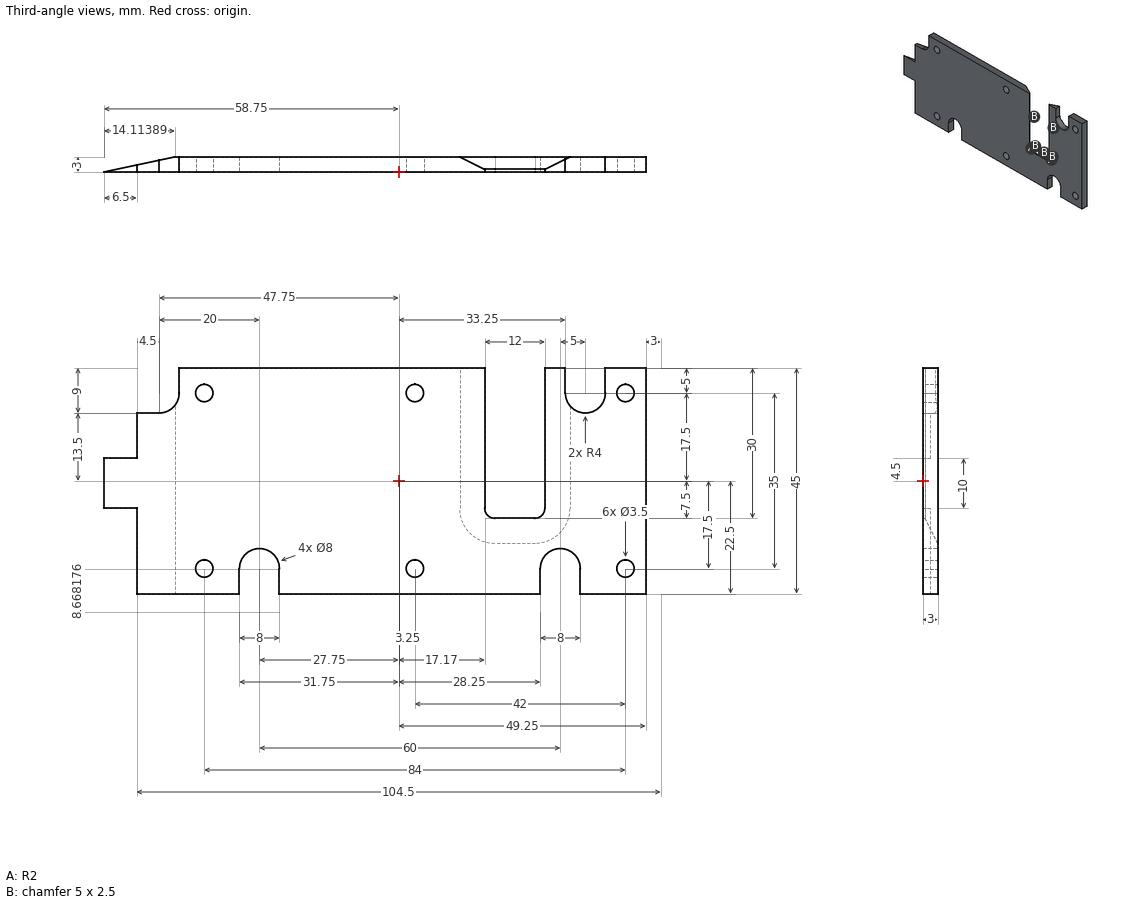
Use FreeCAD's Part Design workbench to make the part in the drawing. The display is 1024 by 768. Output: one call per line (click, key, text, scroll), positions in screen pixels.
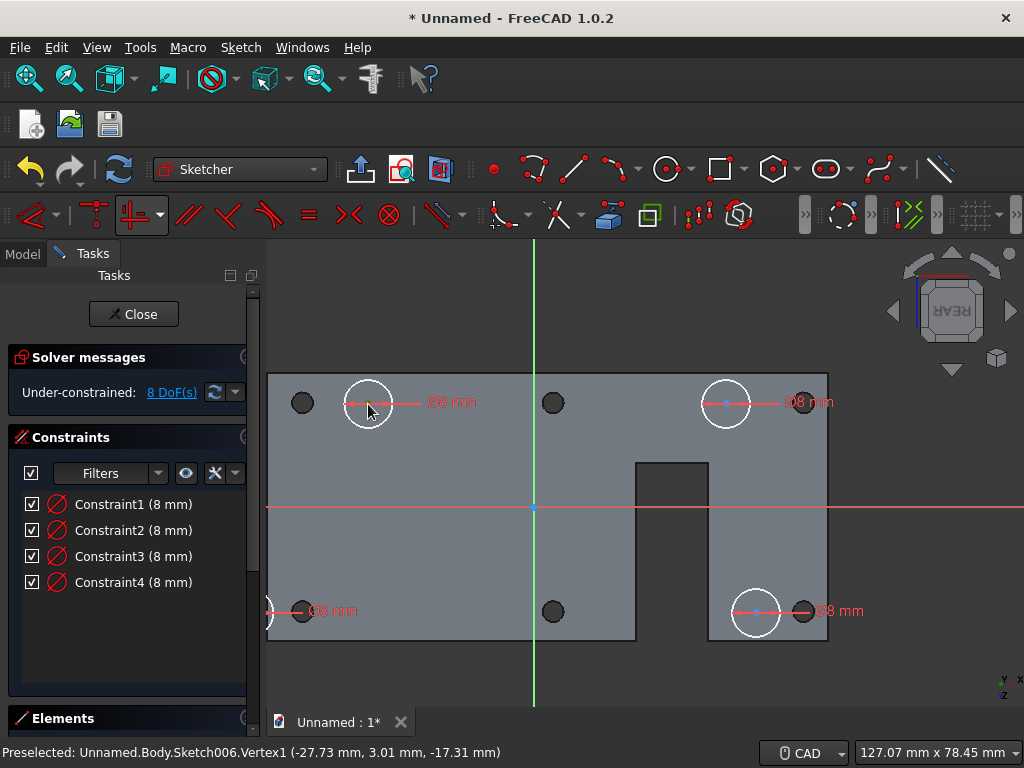
click(726, 404)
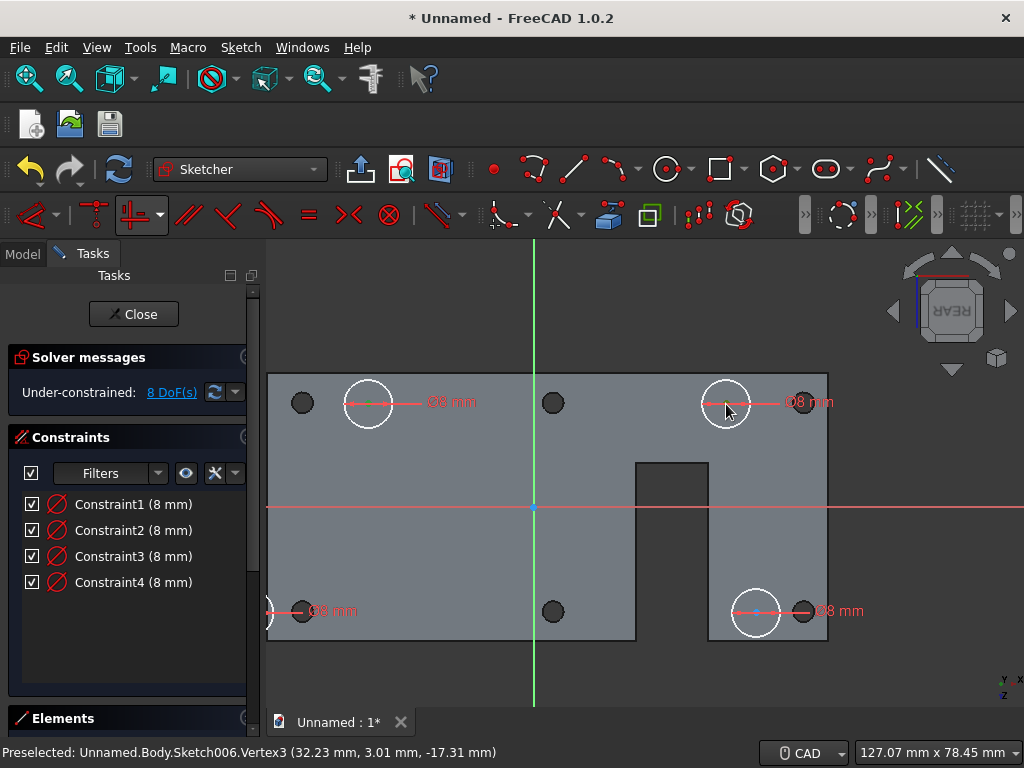
click(162, 216)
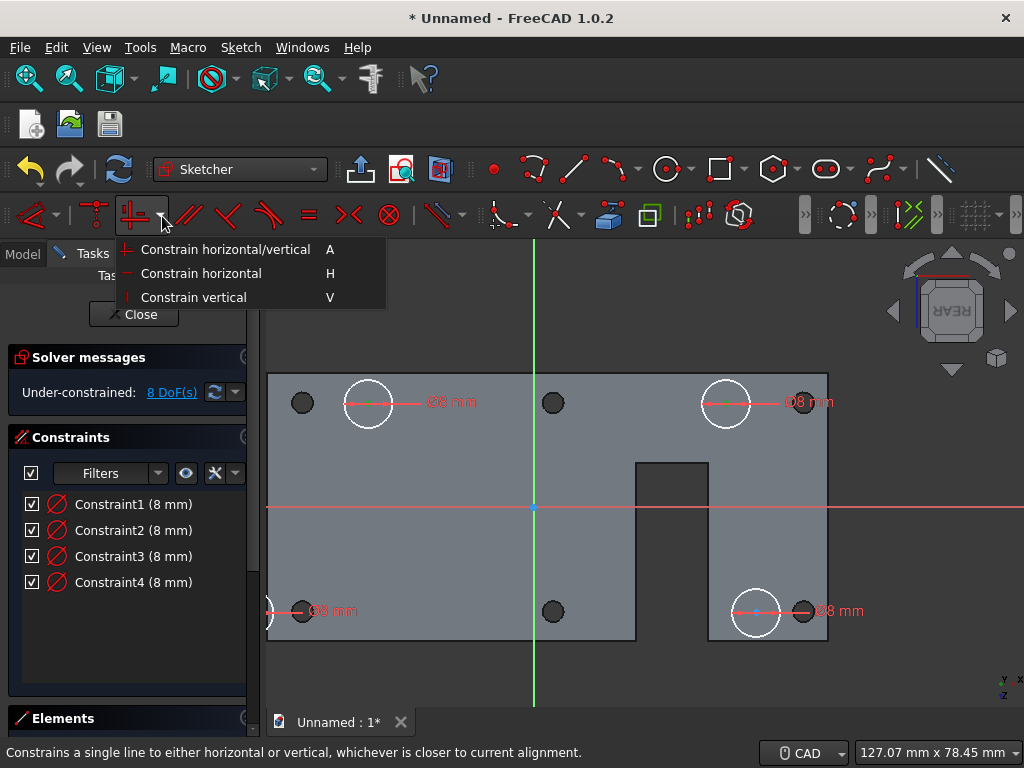
click(251, 273)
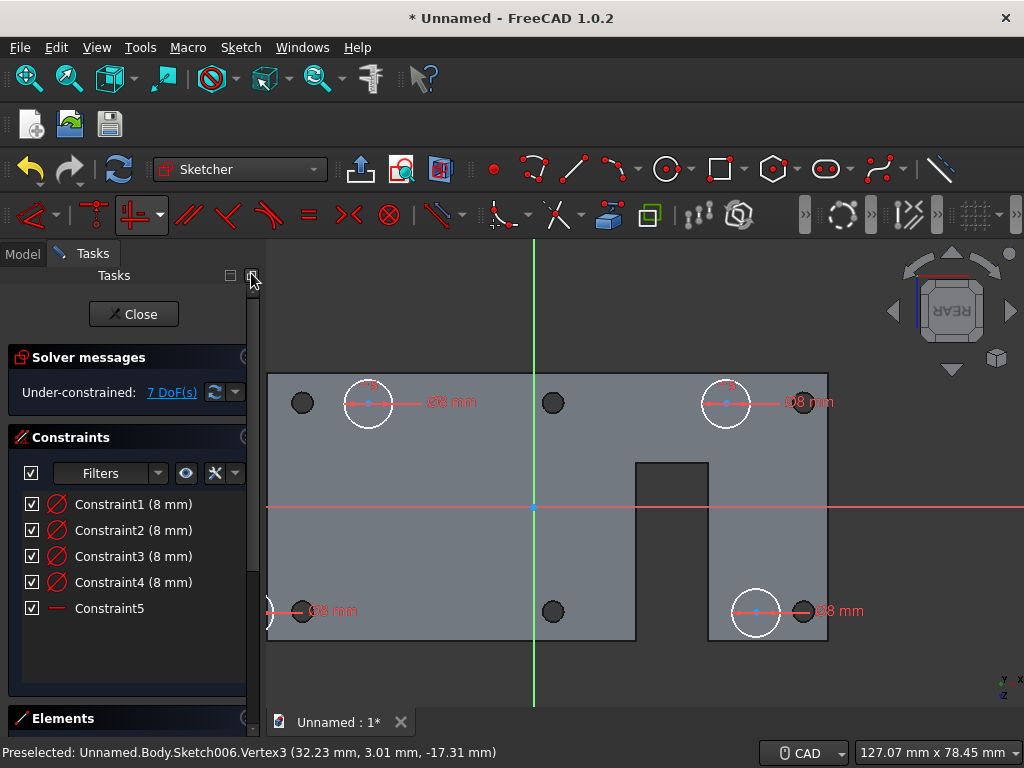
scroll(727, 403, down, 2)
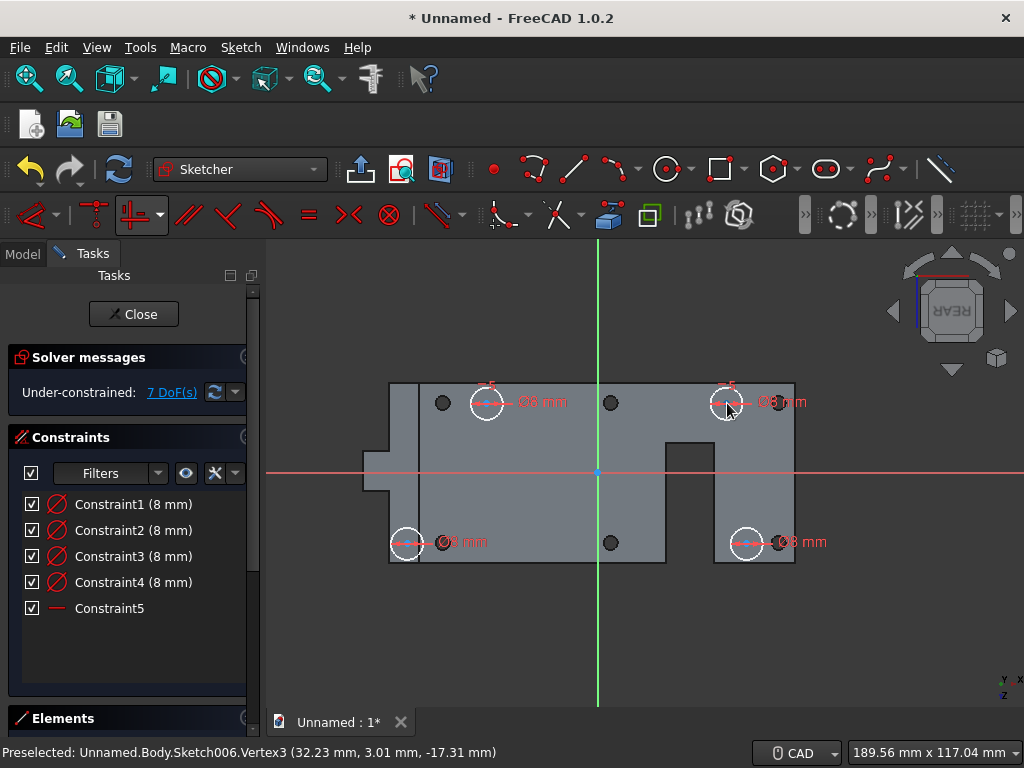
click(407, 544)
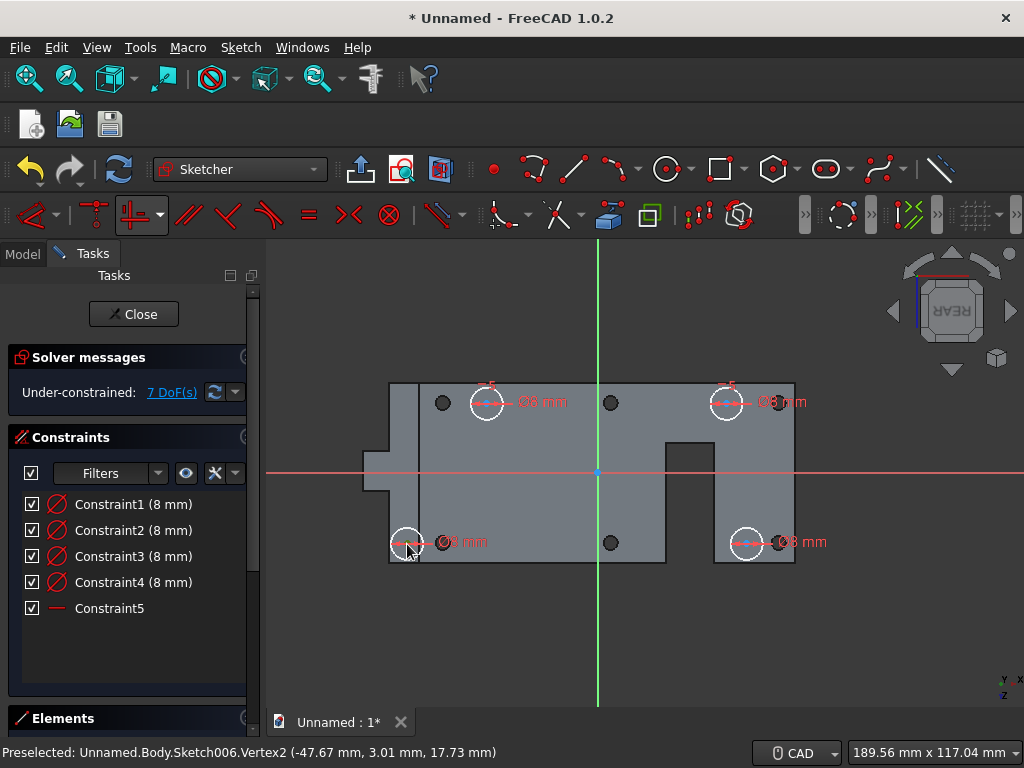
click(747, 544)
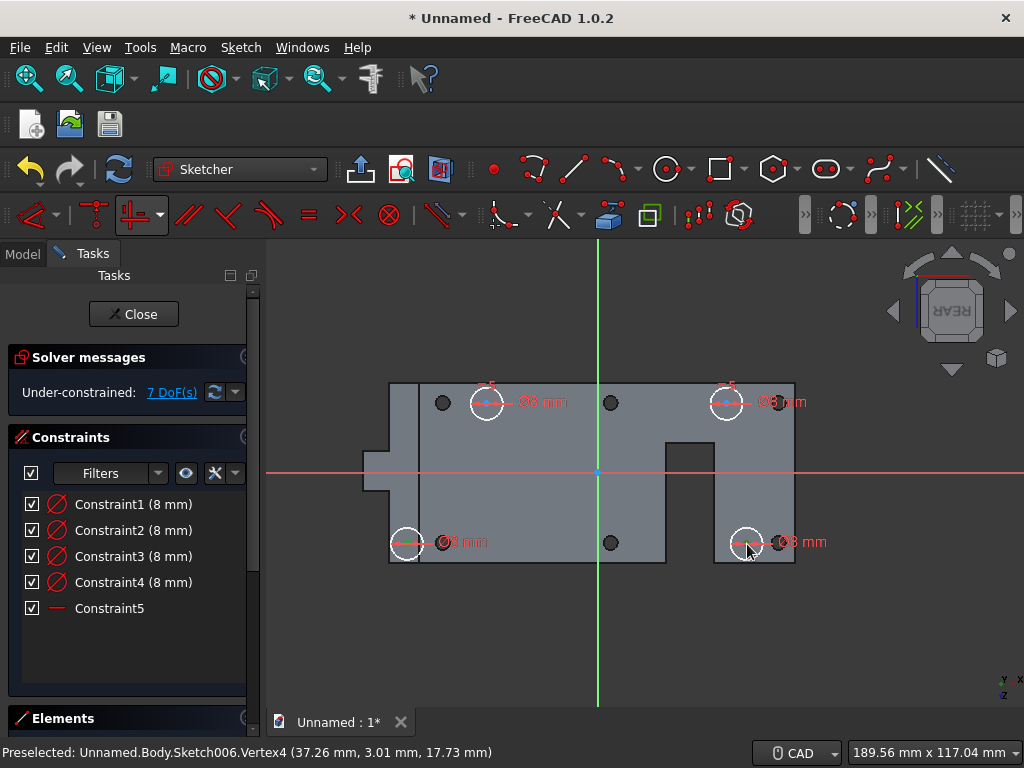
click(162, 216)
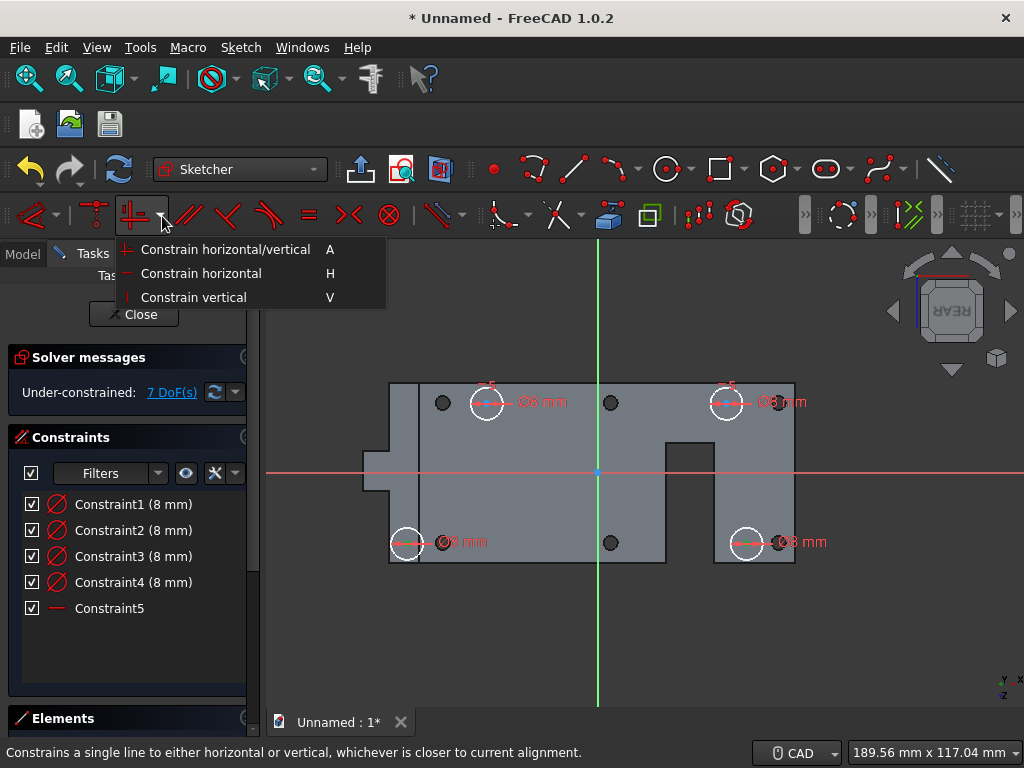
click(251, 273)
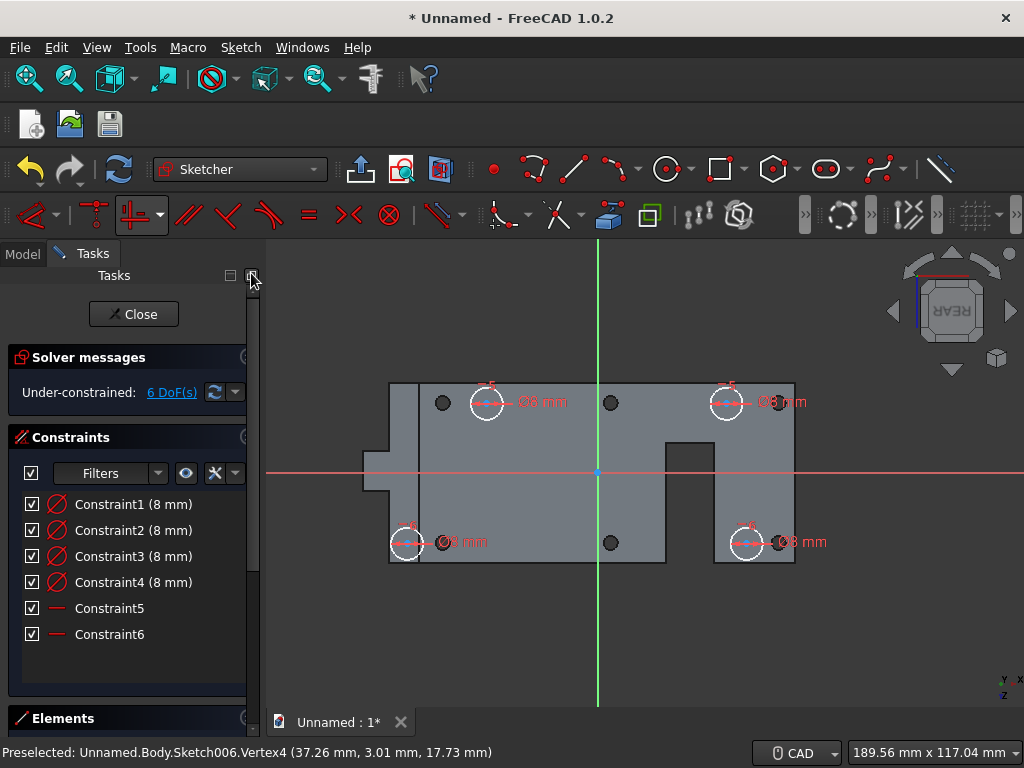
click(32, 216)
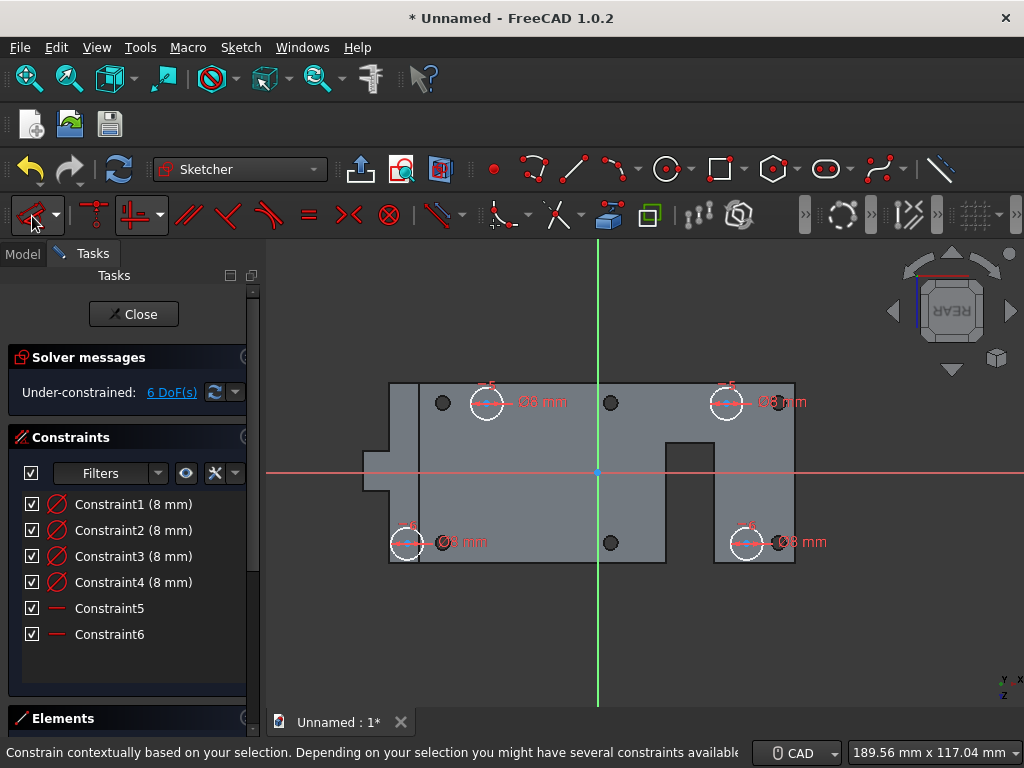
scroll(727, 404, up, 4)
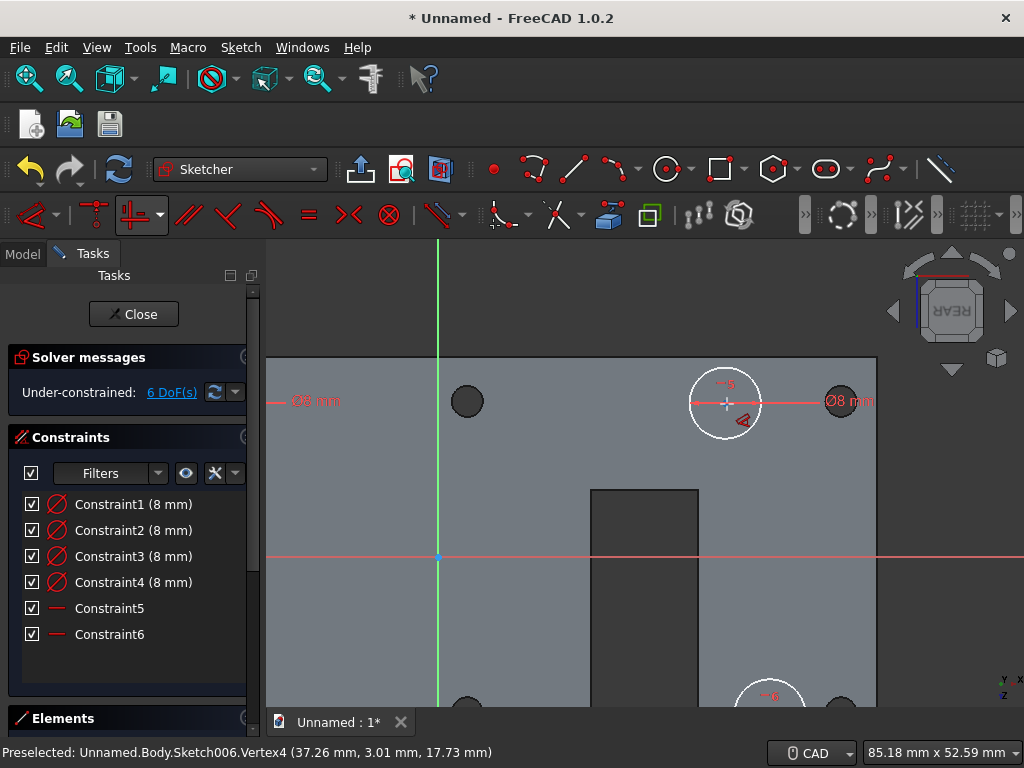
click(725, 403)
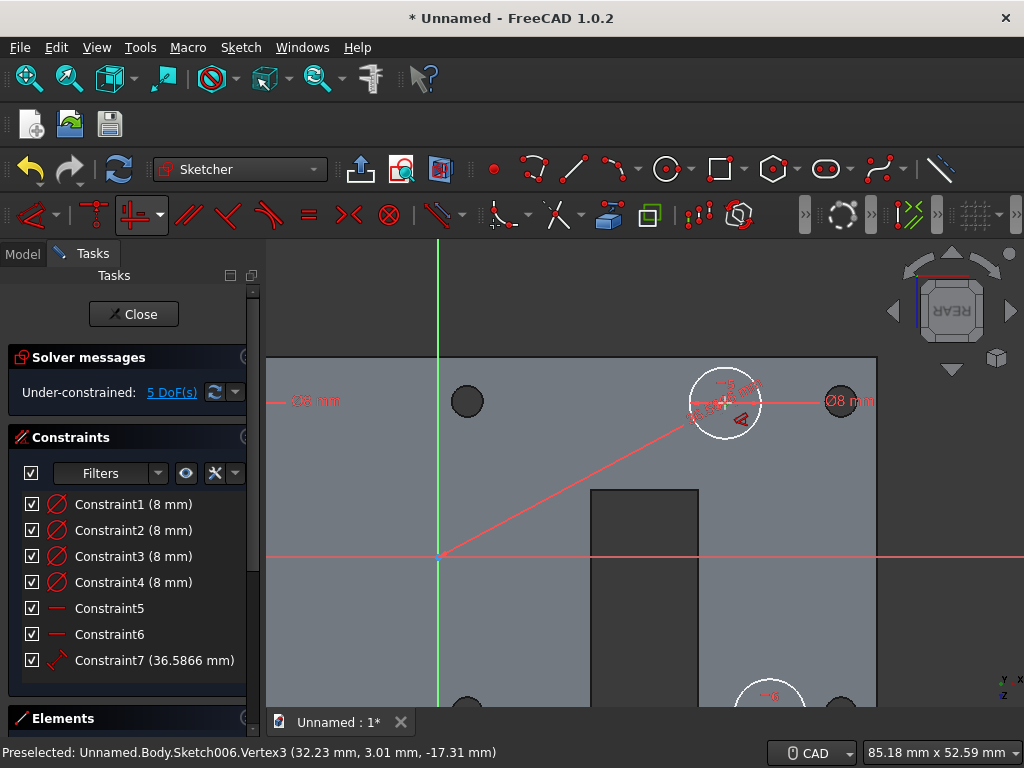
scroll(727, 404, down, 4)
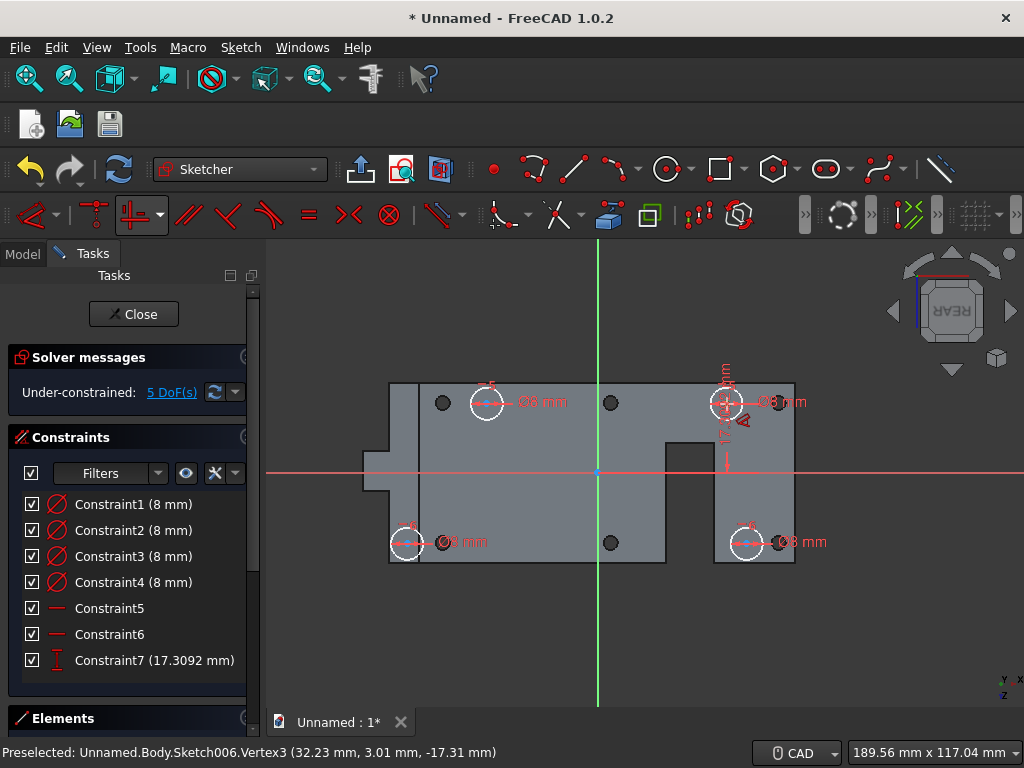
scroll(747, 544, up, 4)